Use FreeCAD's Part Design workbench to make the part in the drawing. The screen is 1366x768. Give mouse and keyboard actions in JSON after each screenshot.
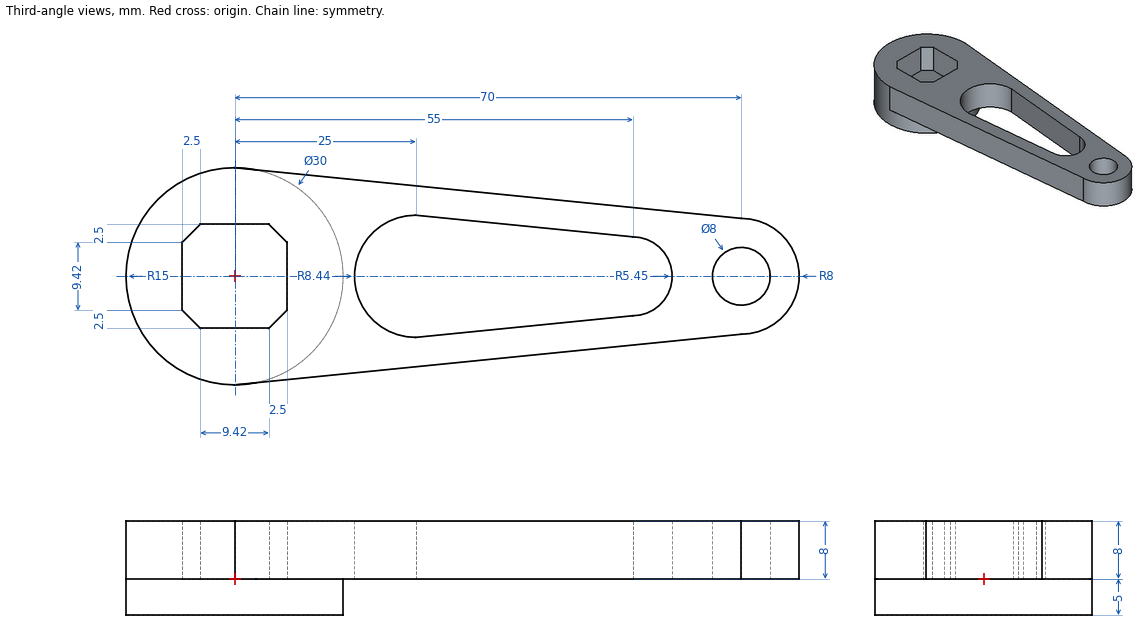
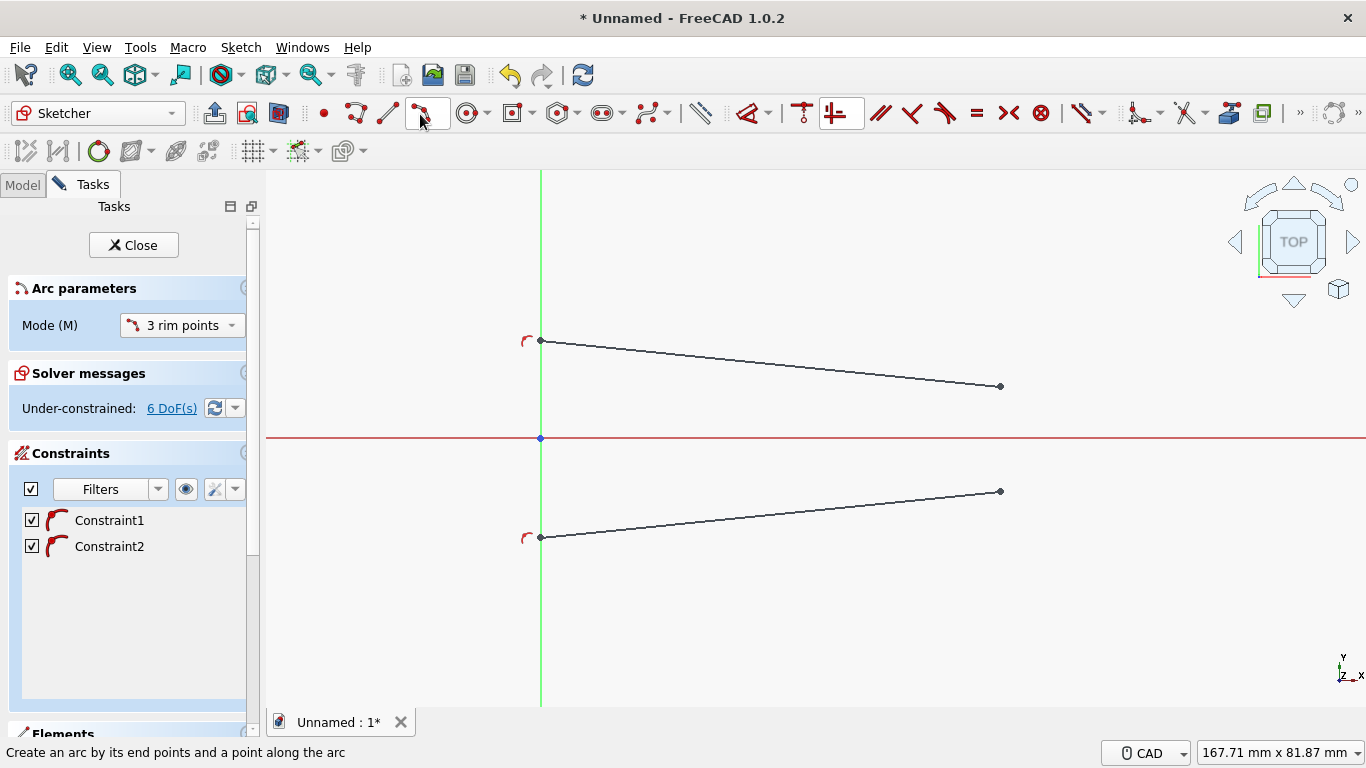
{"action": "left_click", "coordinate": [541, 341]}
{"action": "left_click", "coordinate": [541, 538]}
{"action": "left_click", "coordinate": [447, 408]}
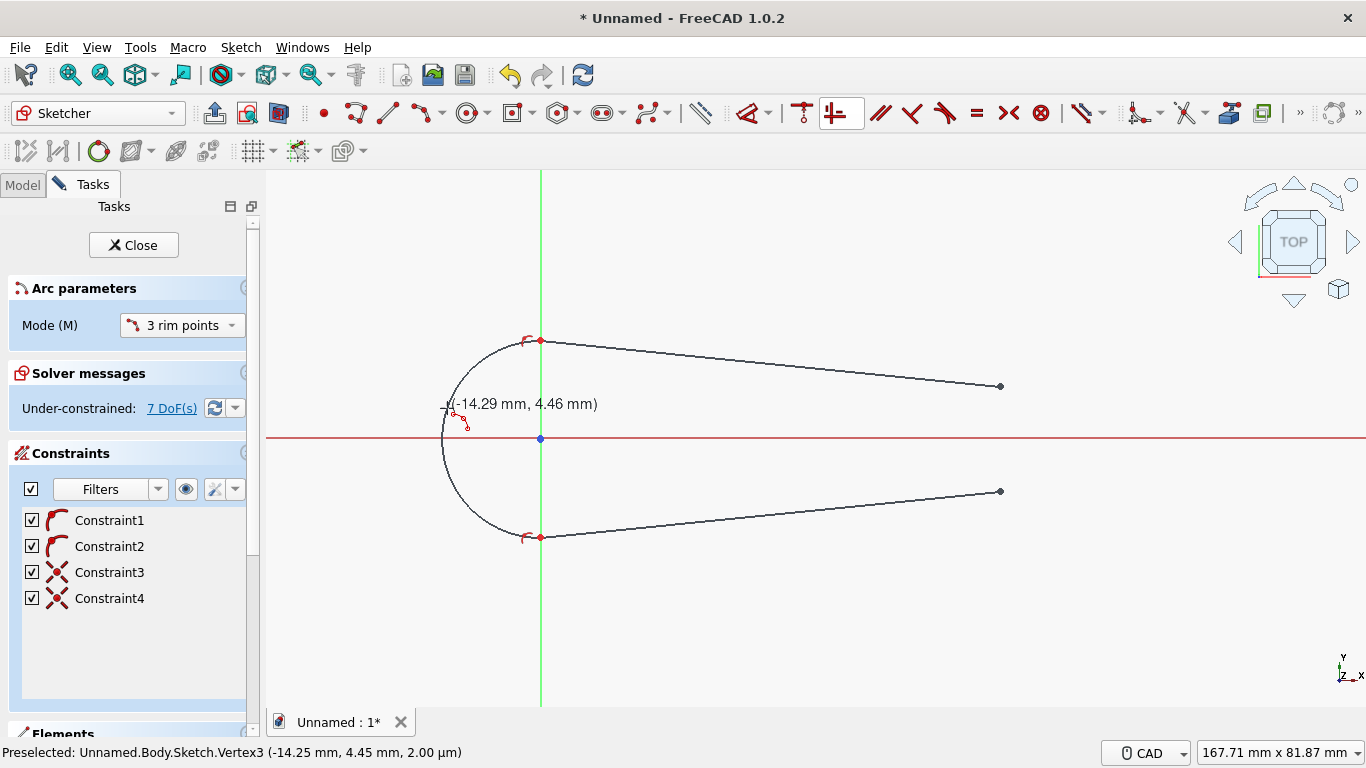
{"action": "left_click", "coordinate": [1000, 492]}
{"action": "left_click", "coordinate": [1000, 387]}
{"action": "left_click", "coordinate": [1050, 454]}
{"action": "key", "text": "Escape"}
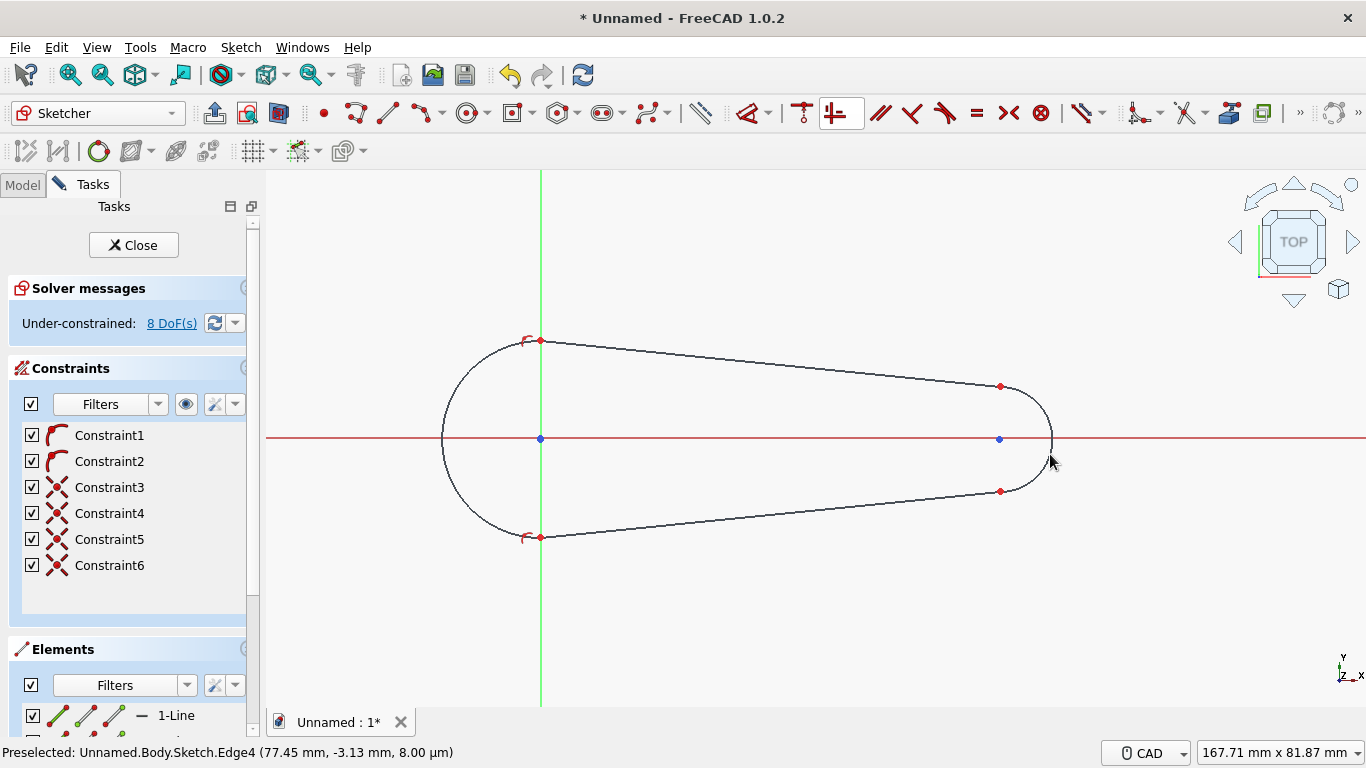
{"action": "left_click_drag", "start_coordinate": [531, 428], "coordinate": [551, 449]}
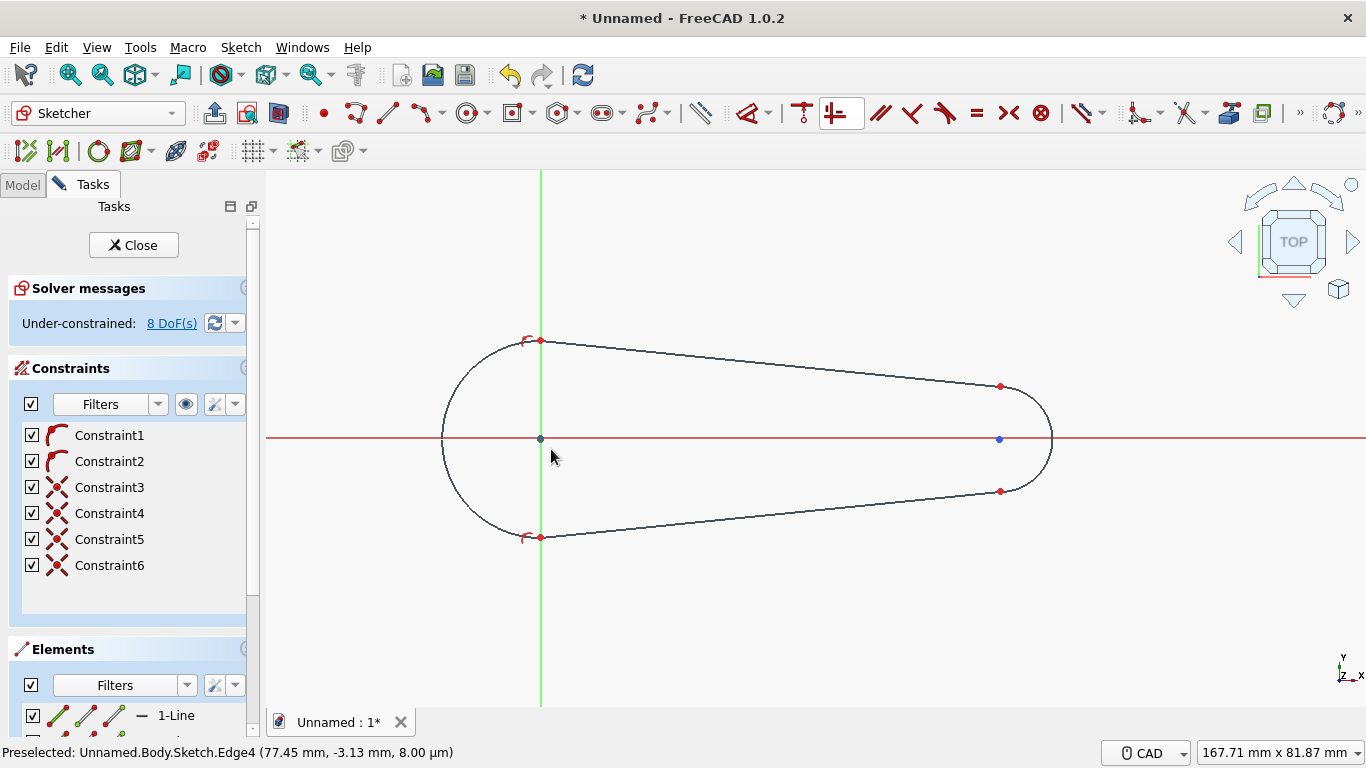
{"action": "left_click", "coordinate": [802, 114]}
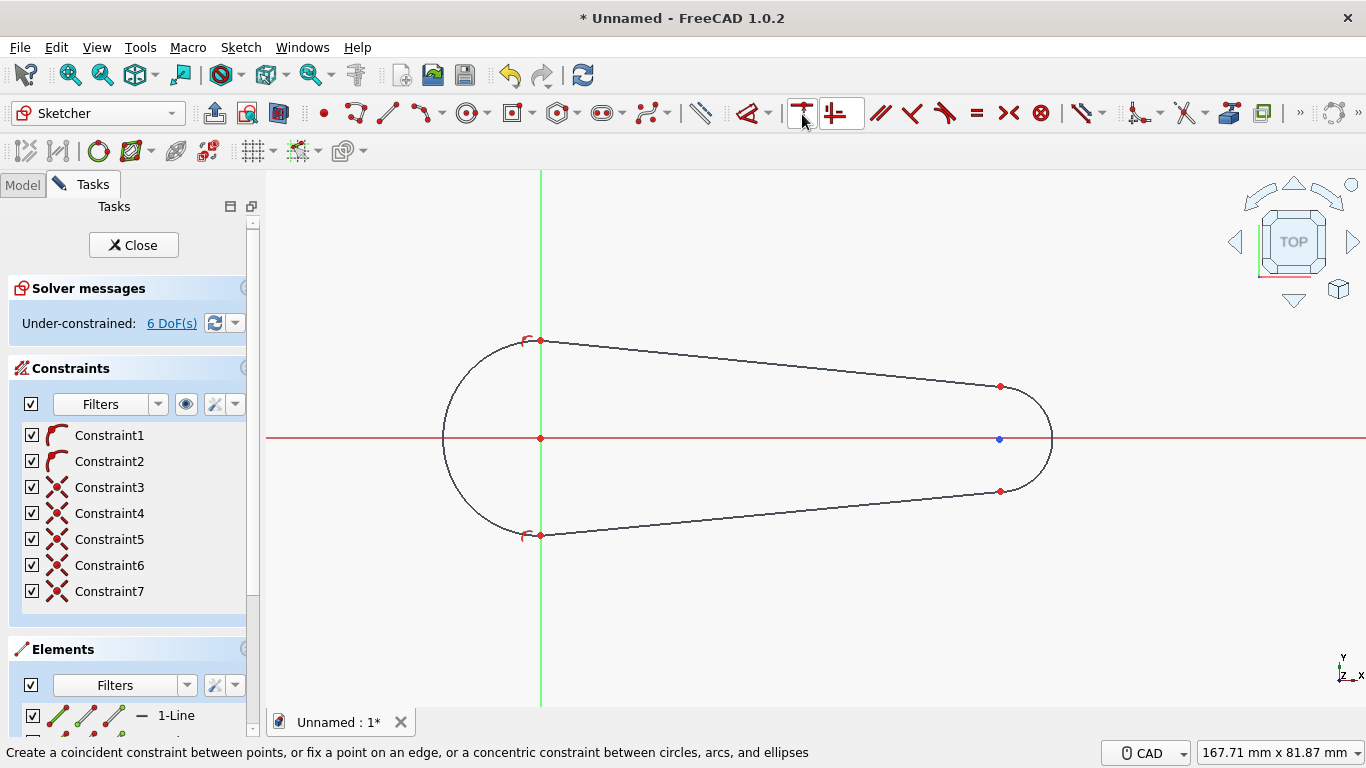
{"action": "left_click", "coordinate": [1000, 439]}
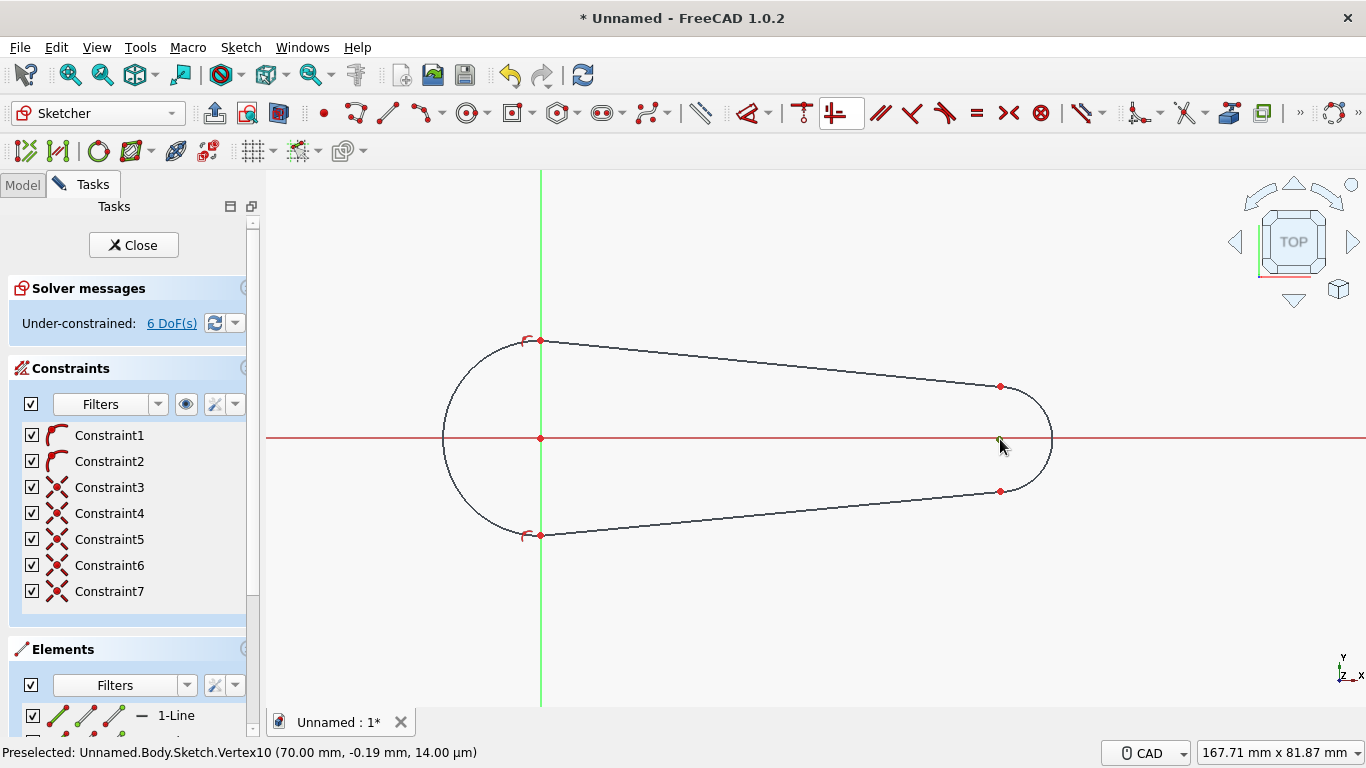
{"action": "left_click", "coordinate": [359, 438]}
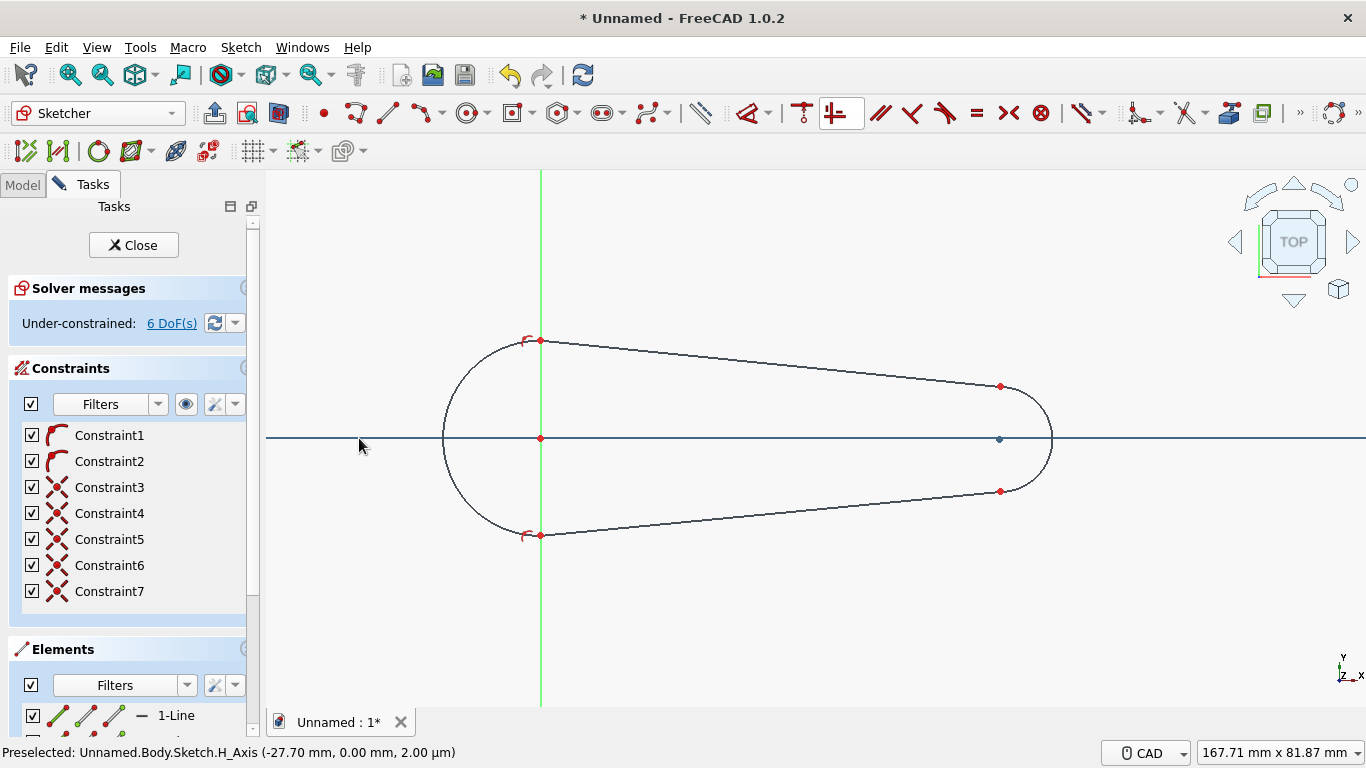
{"action": "left_click", "coordinate": [802, 114]}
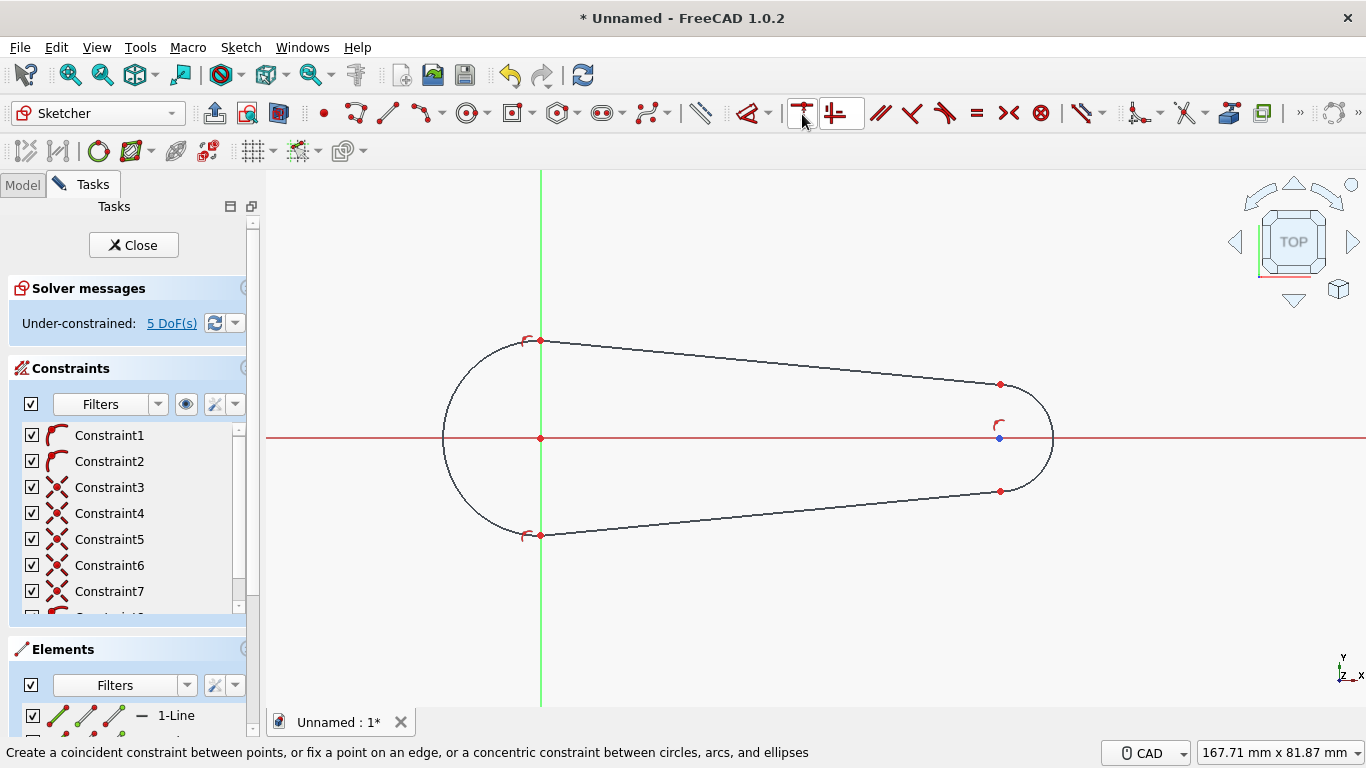
{"action": "key", "text": "d"}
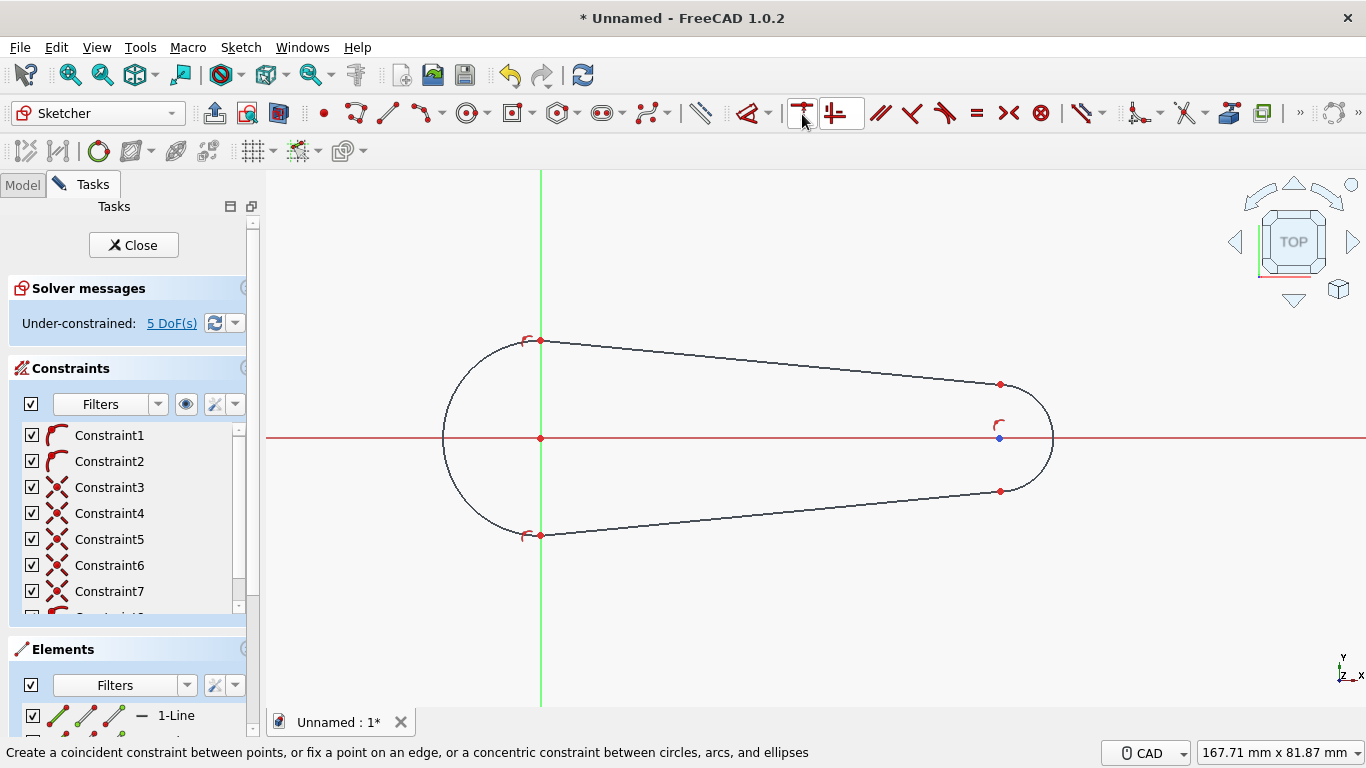
{"action": "left_click", "coordinate": [462, 381]}
{"action": "left_click", "coordinate": [436, 362]}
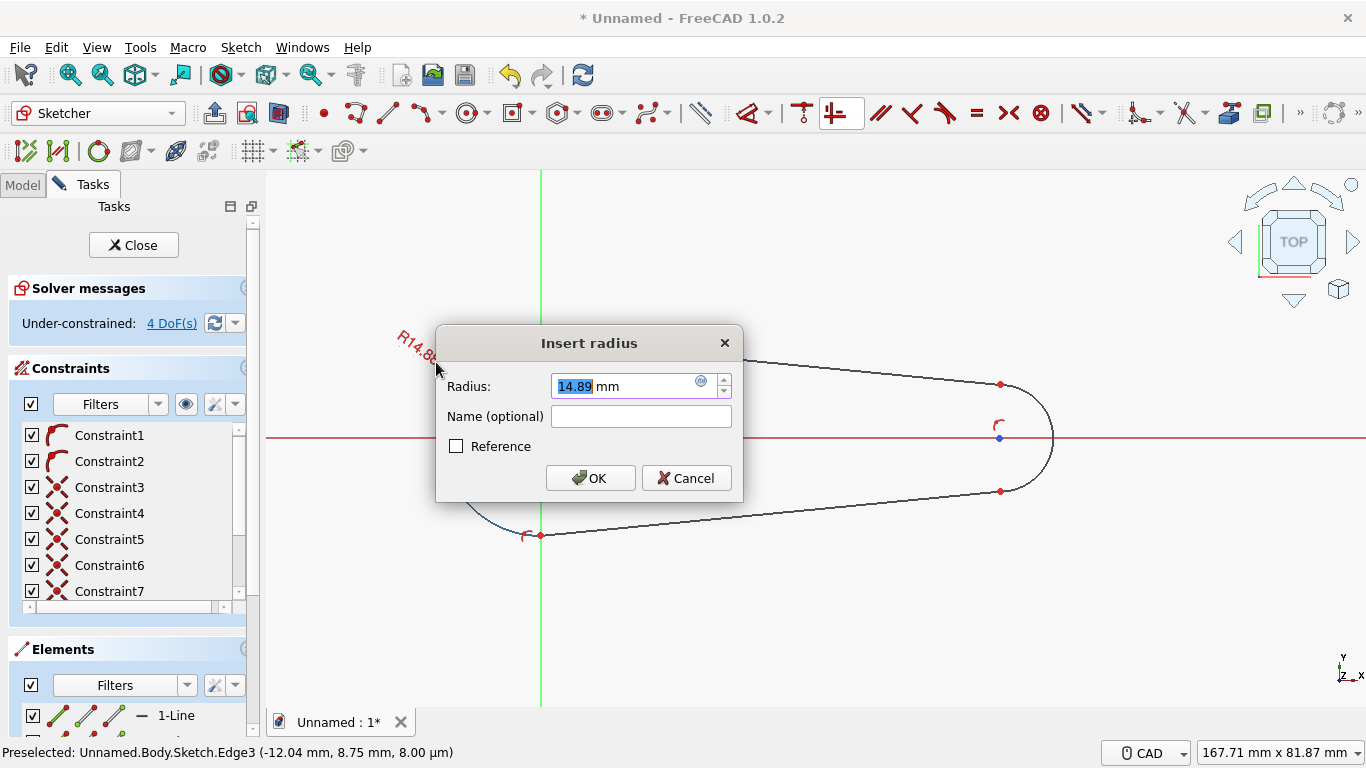
{"action": "type", "text": "15"}
{"action": "key", "text": "Return"}